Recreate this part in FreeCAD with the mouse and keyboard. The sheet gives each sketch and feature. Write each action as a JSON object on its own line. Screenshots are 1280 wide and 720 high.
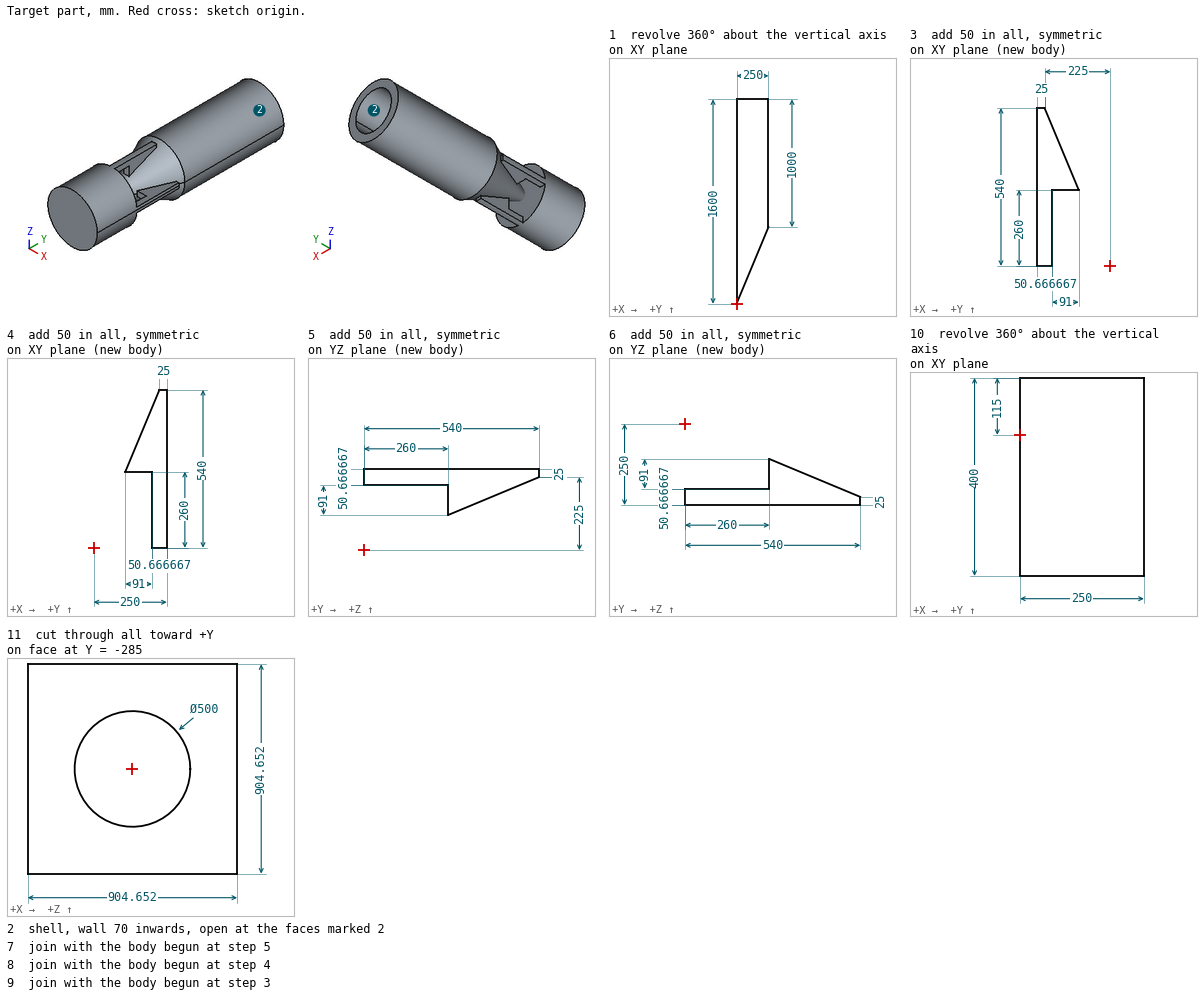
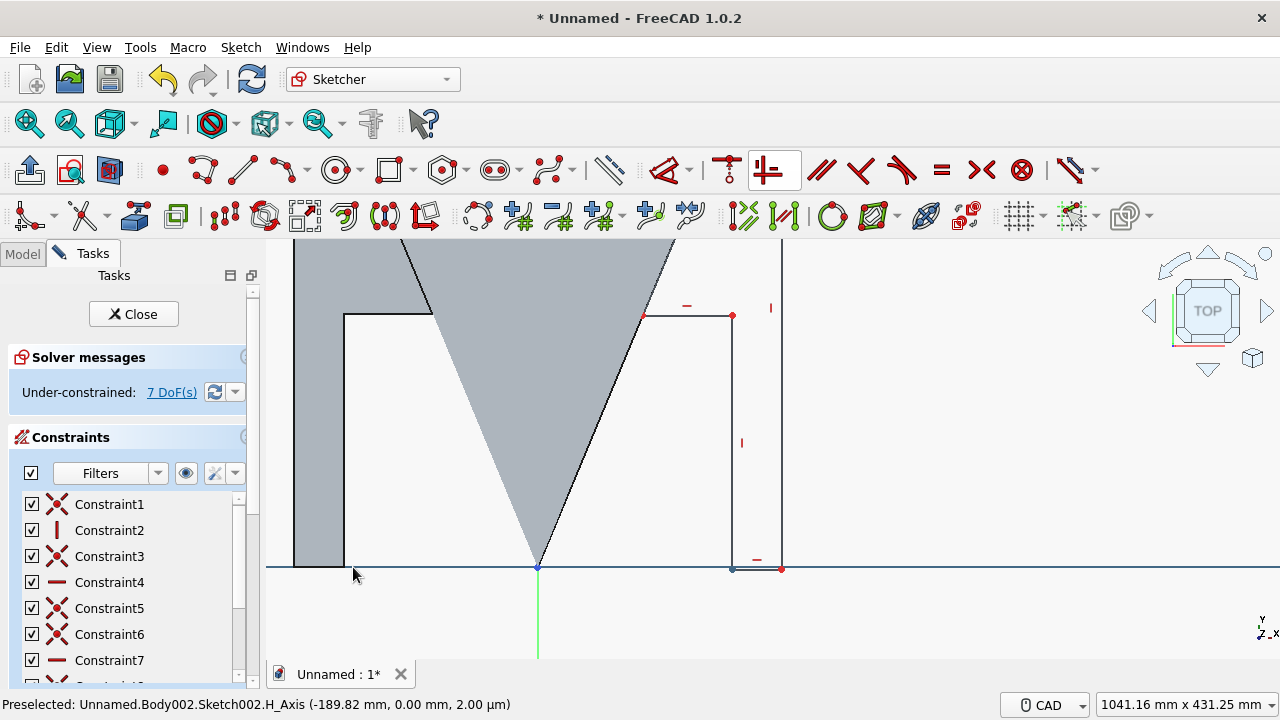
{"action": "left_click", "coordinate": [728, 170]}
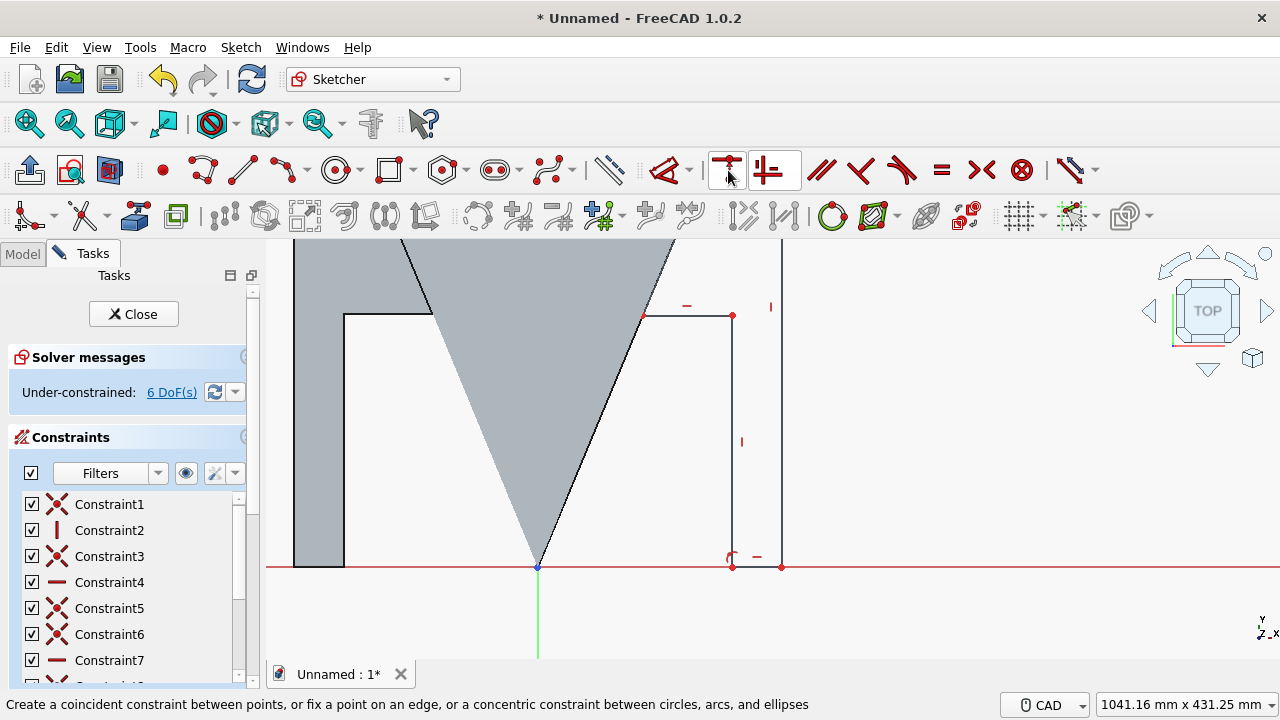
{"action": "left_click", "coordinate": [664, 170]}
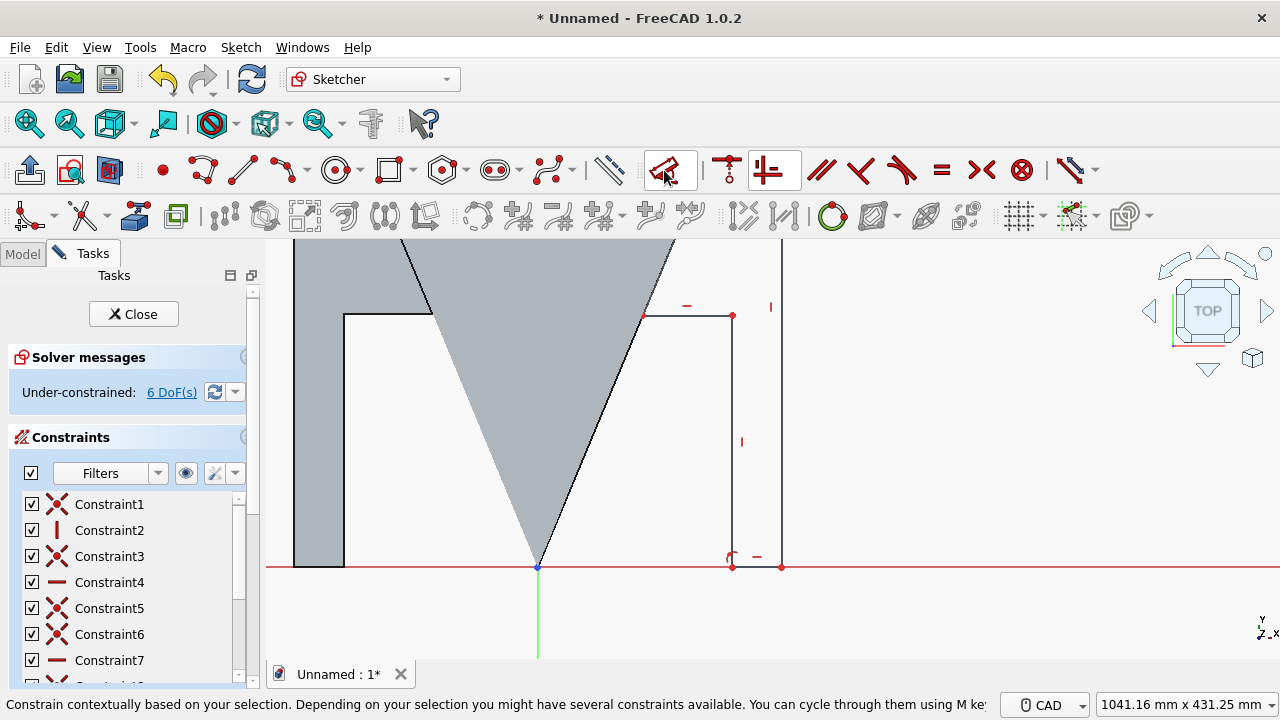
{"action": "scroll", "coordinate": [741, 567], "scroll_direction": "down", "scroll_amount": 4}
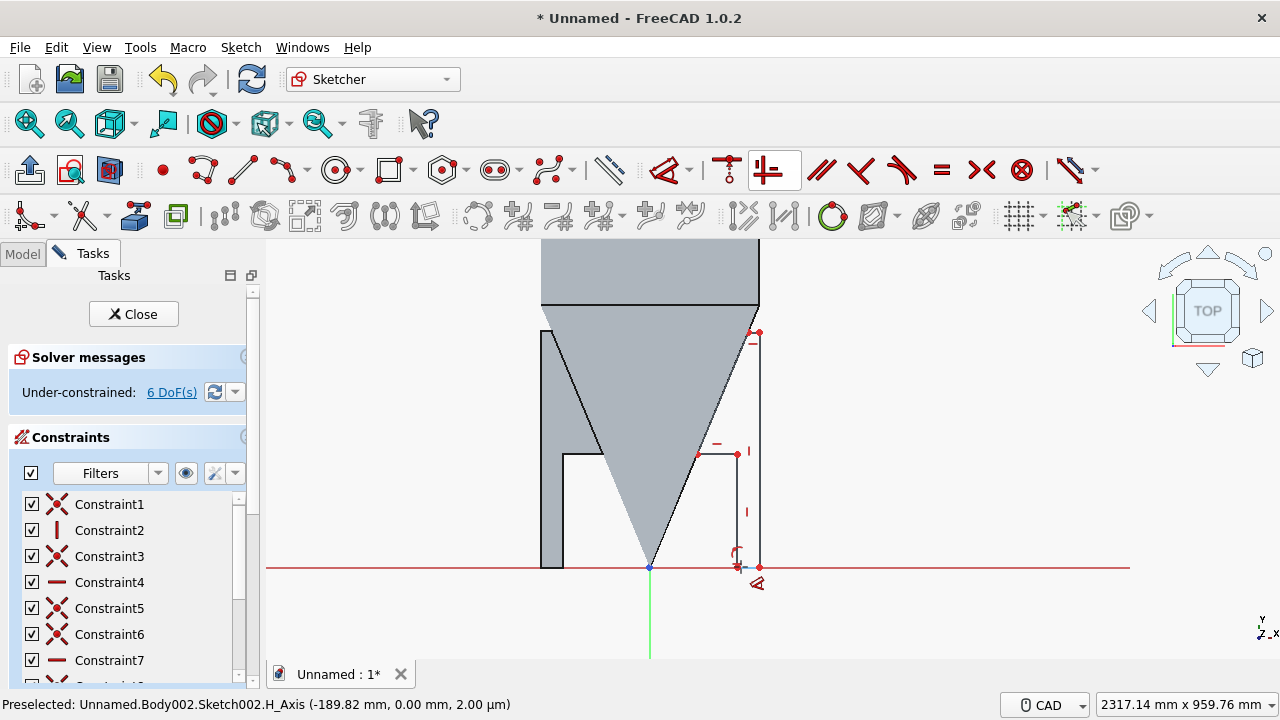
{"action": "scroll", "coordinate": [755, 333], "scroll_direction": "up", "scroll_amount": 7}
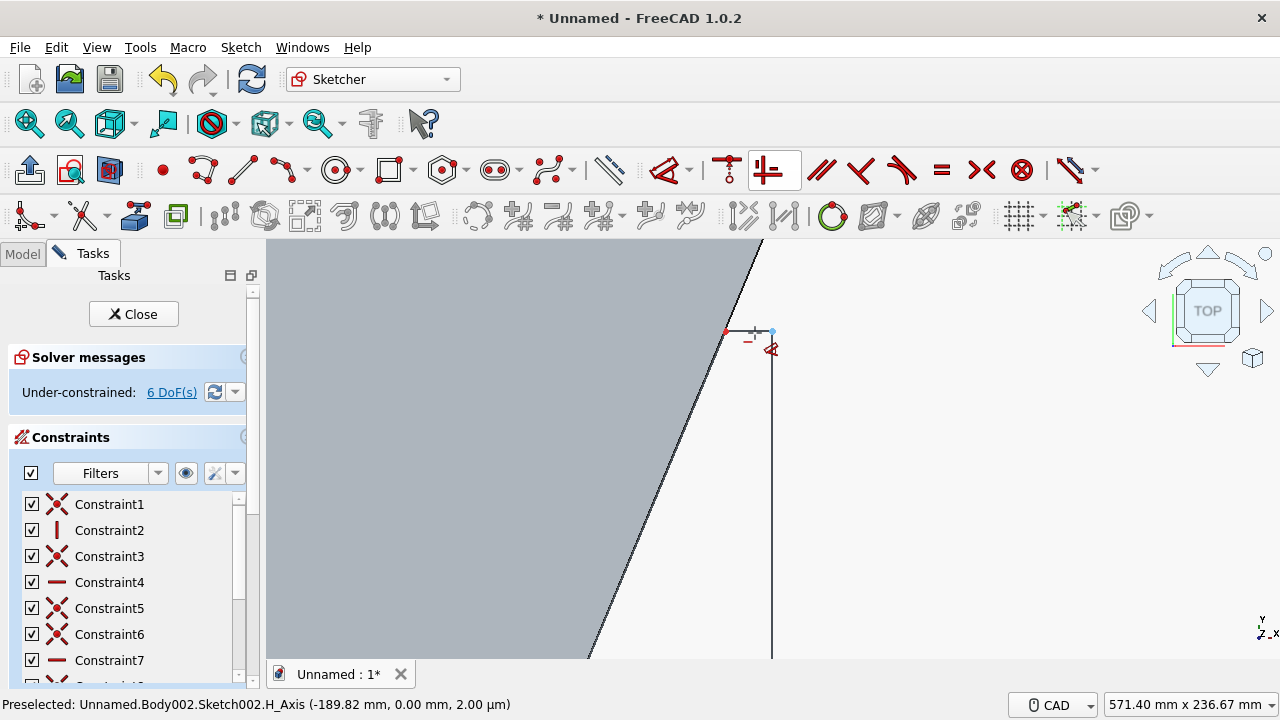
{"action": "left_click", "coordinate": [754, 331]}
{"action": "left_click", "coordinate": [749, 297]}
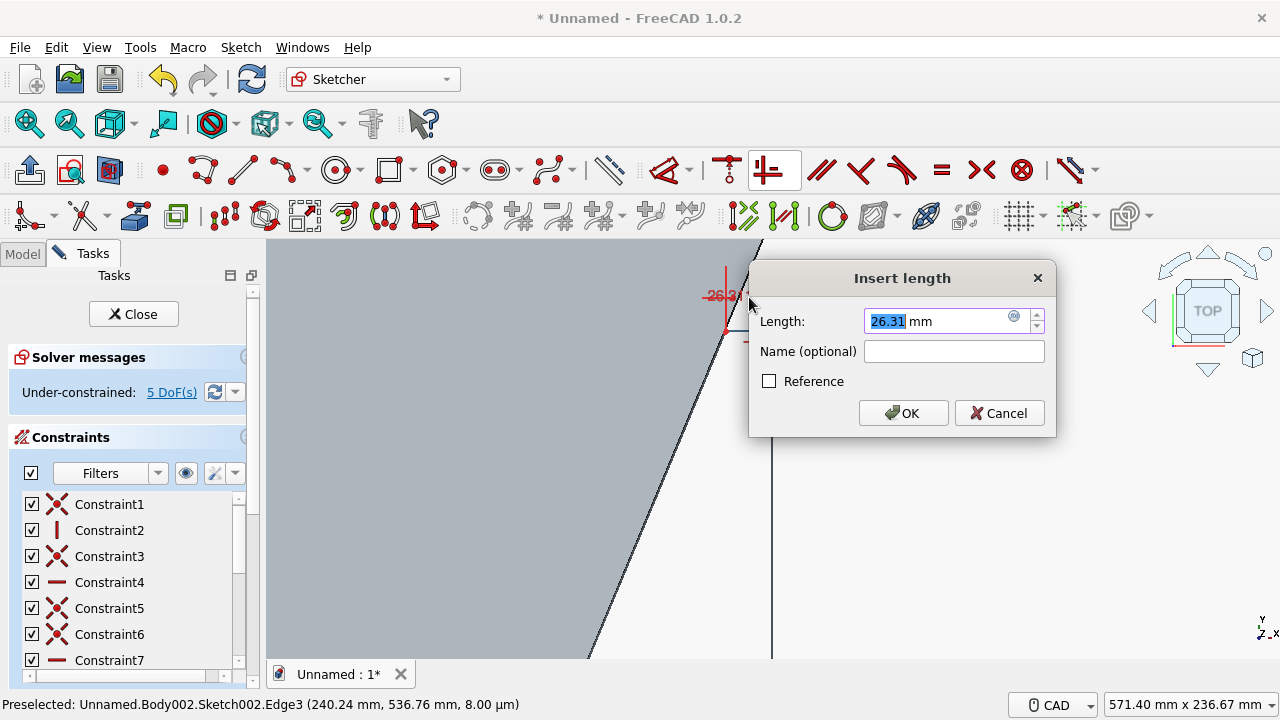
{"action": "type", "text": "25"}
{"action": "key", "text": "Return"}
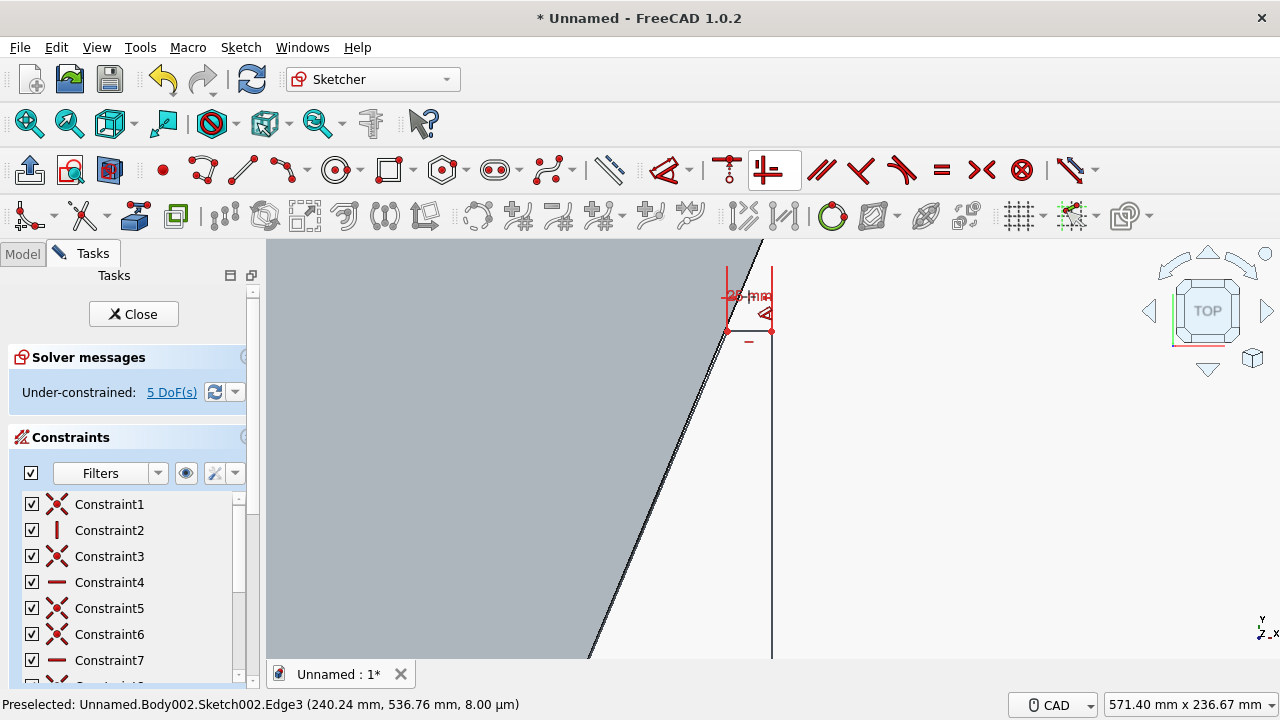
{"action": "scroll", "coordinate": [755, 333], "scroll_direction": "down", "scroll_amount": 7}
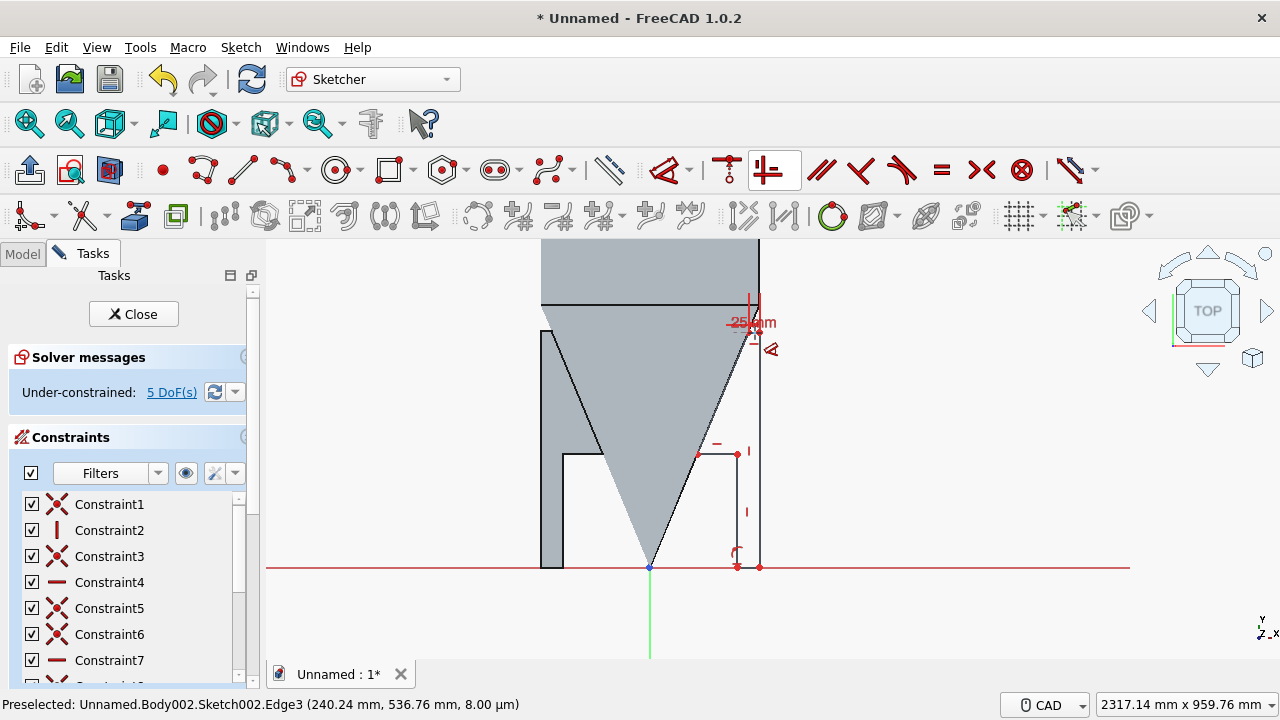
{"action": "scroll", "coordinate": [709, 454], "scroll_direction": "up", "scroll_amount": 2}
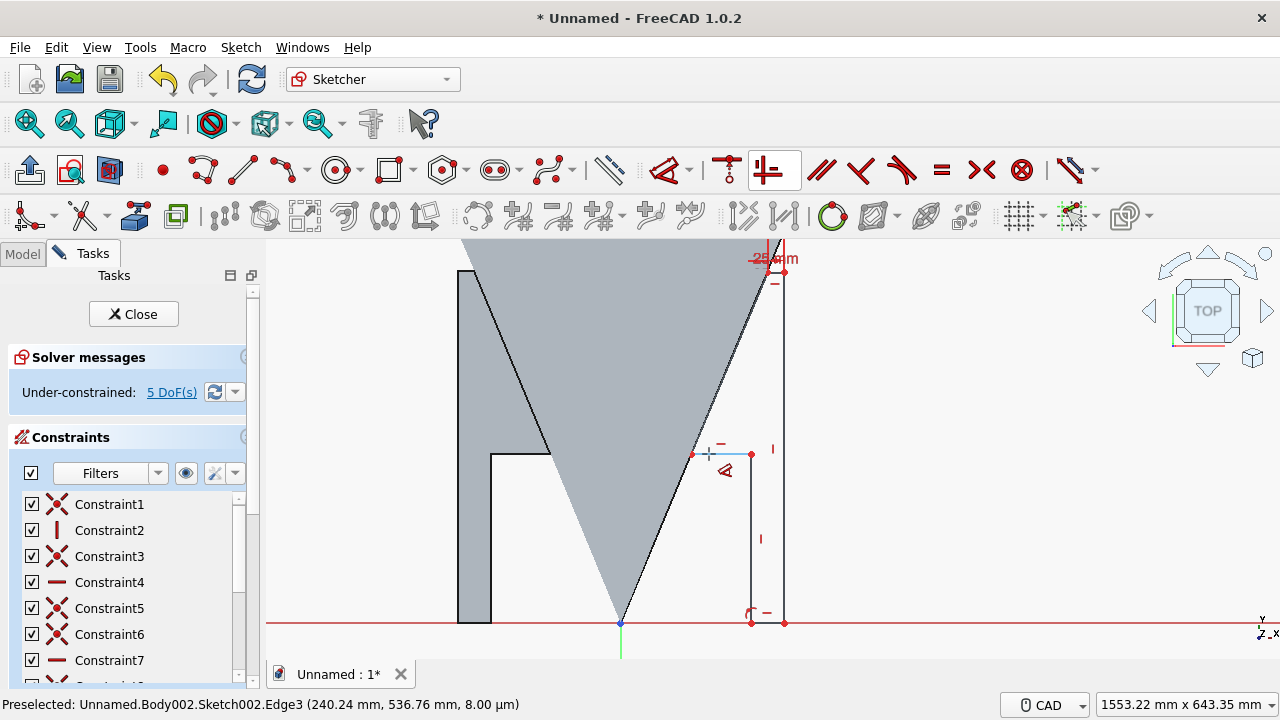
{"action": "left_click", "coordinate": [709, 454]}
{"action": "left_click", "coordinate": [721, 488]}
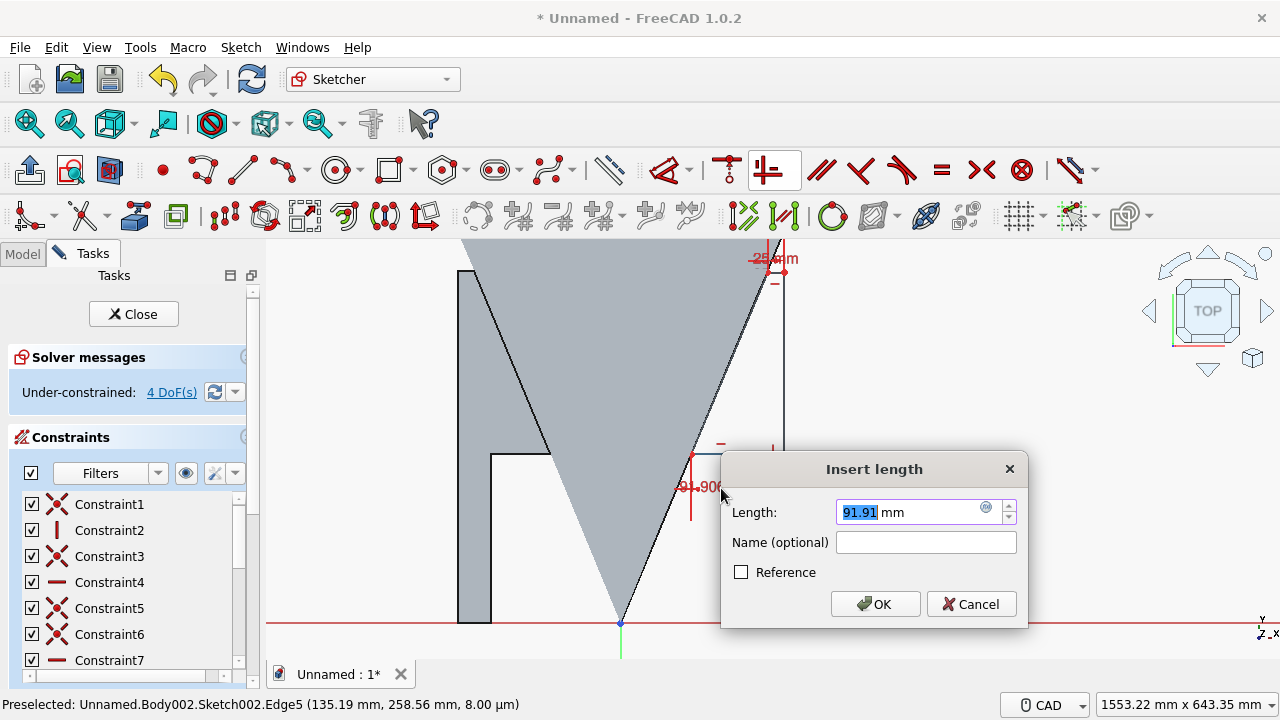
{"action": "type", "text": "91"}
{"action": "key", "text": "Return"}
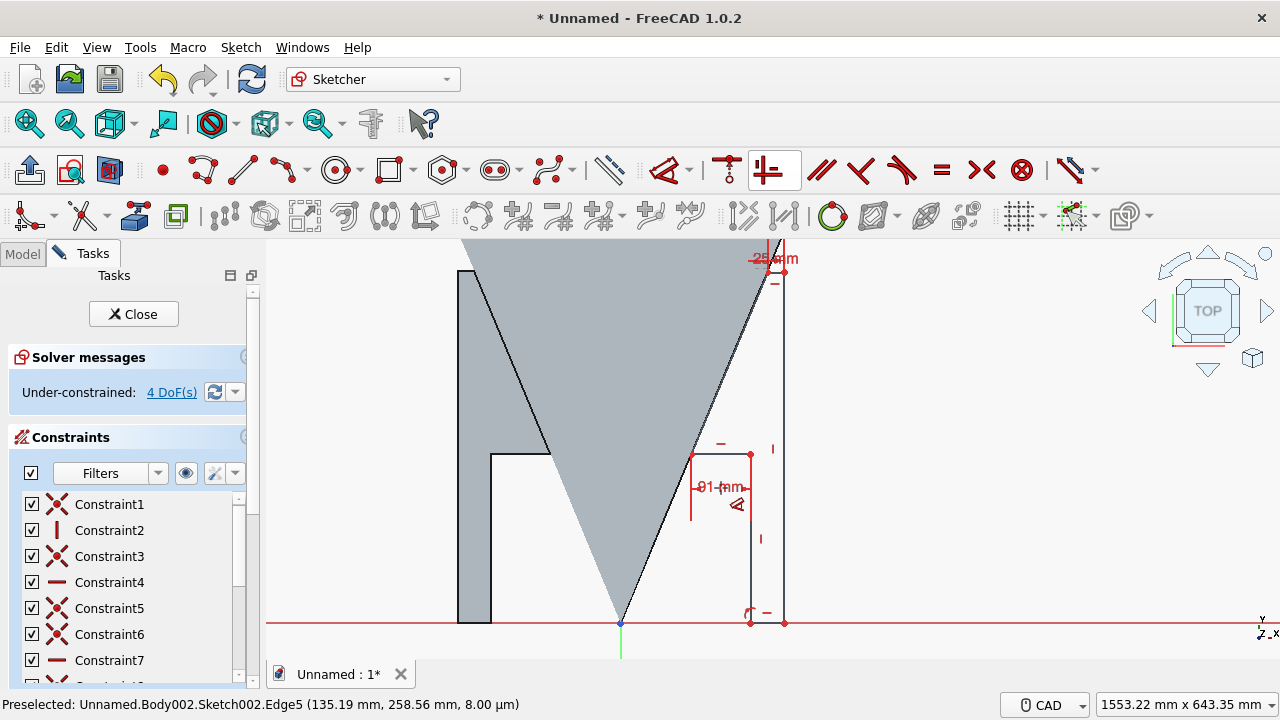
{"action": "left_click", "coordinate": [784, 518]}
{"action": "left_click", "coordinate": [818, 448]}